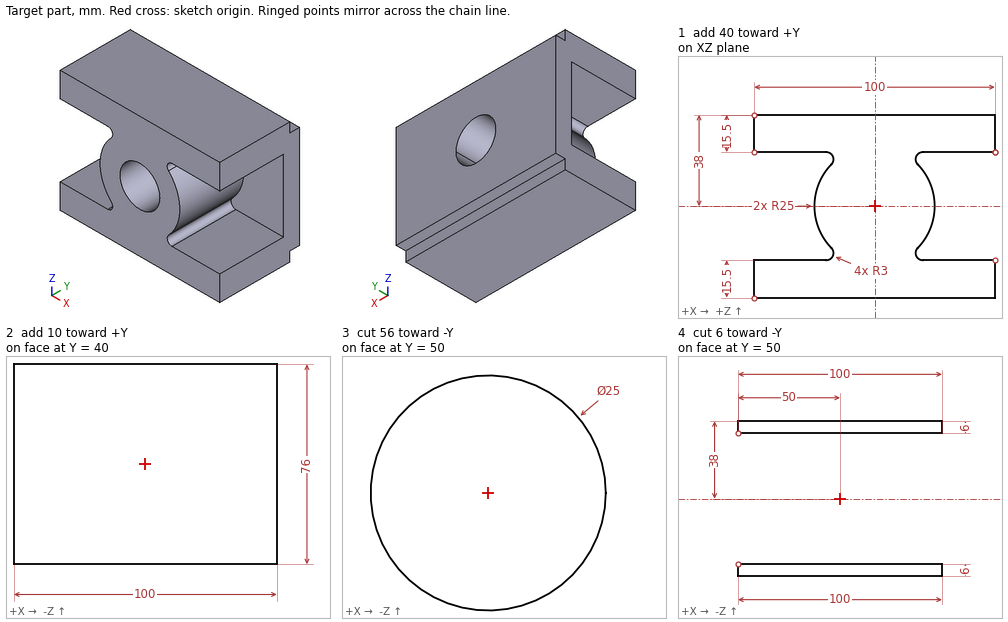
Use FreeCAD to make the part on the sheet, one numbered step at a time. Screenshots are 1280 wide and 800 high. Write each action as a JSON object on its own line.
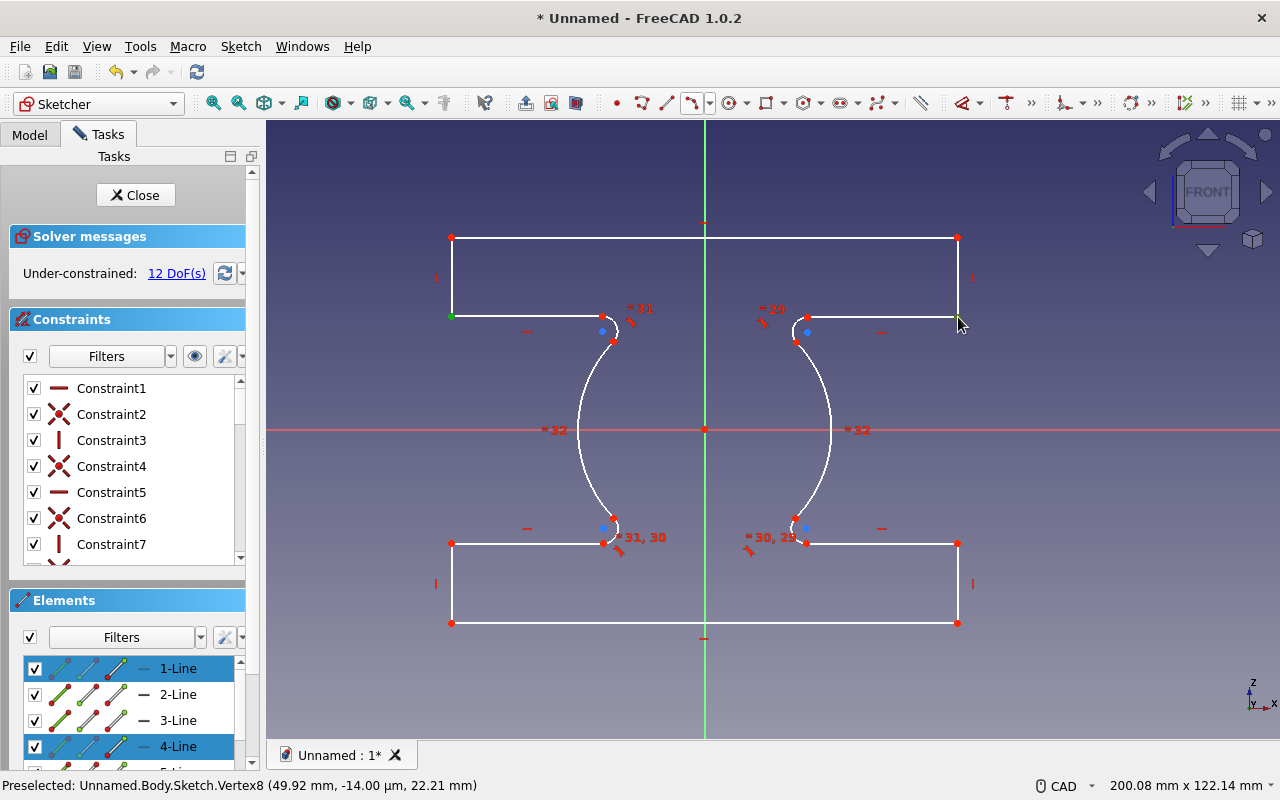
{"action": "left_click", "coordinate": [705, 671]}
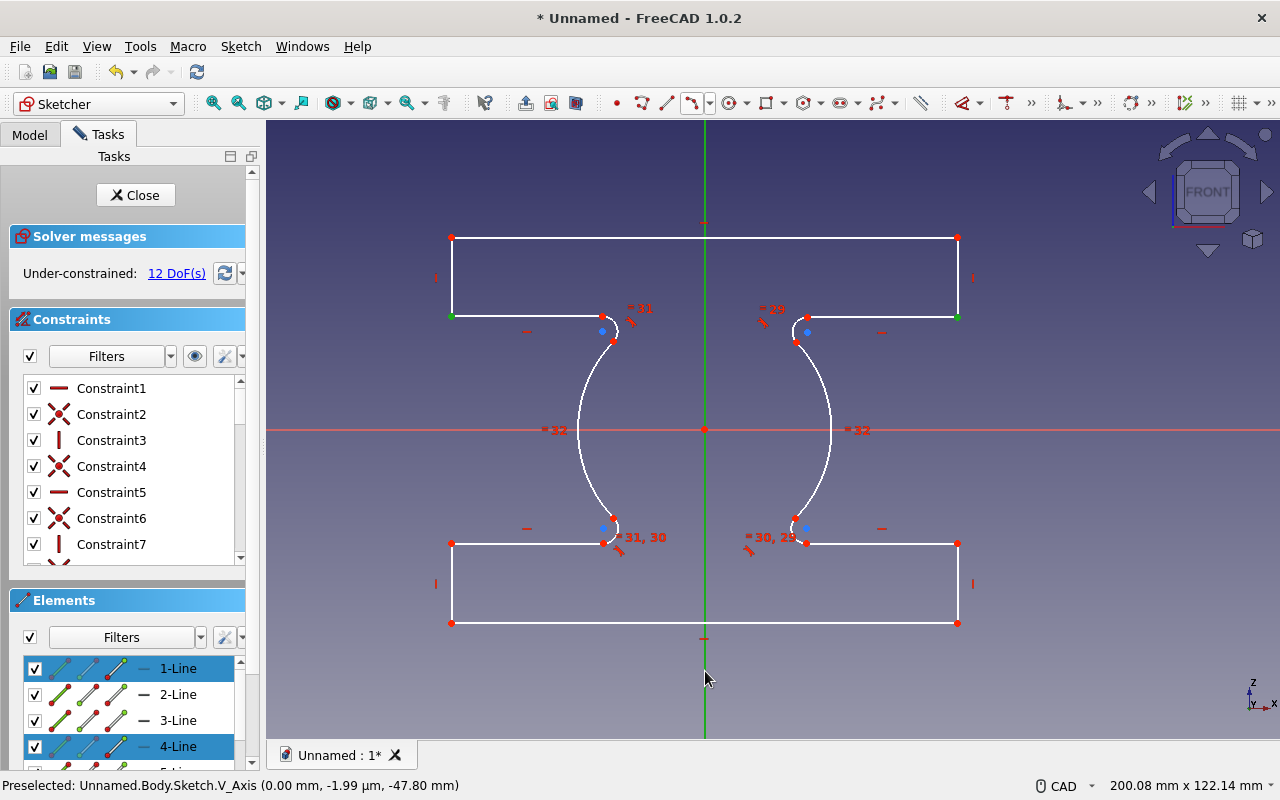
{"action": "key", "text": "s"}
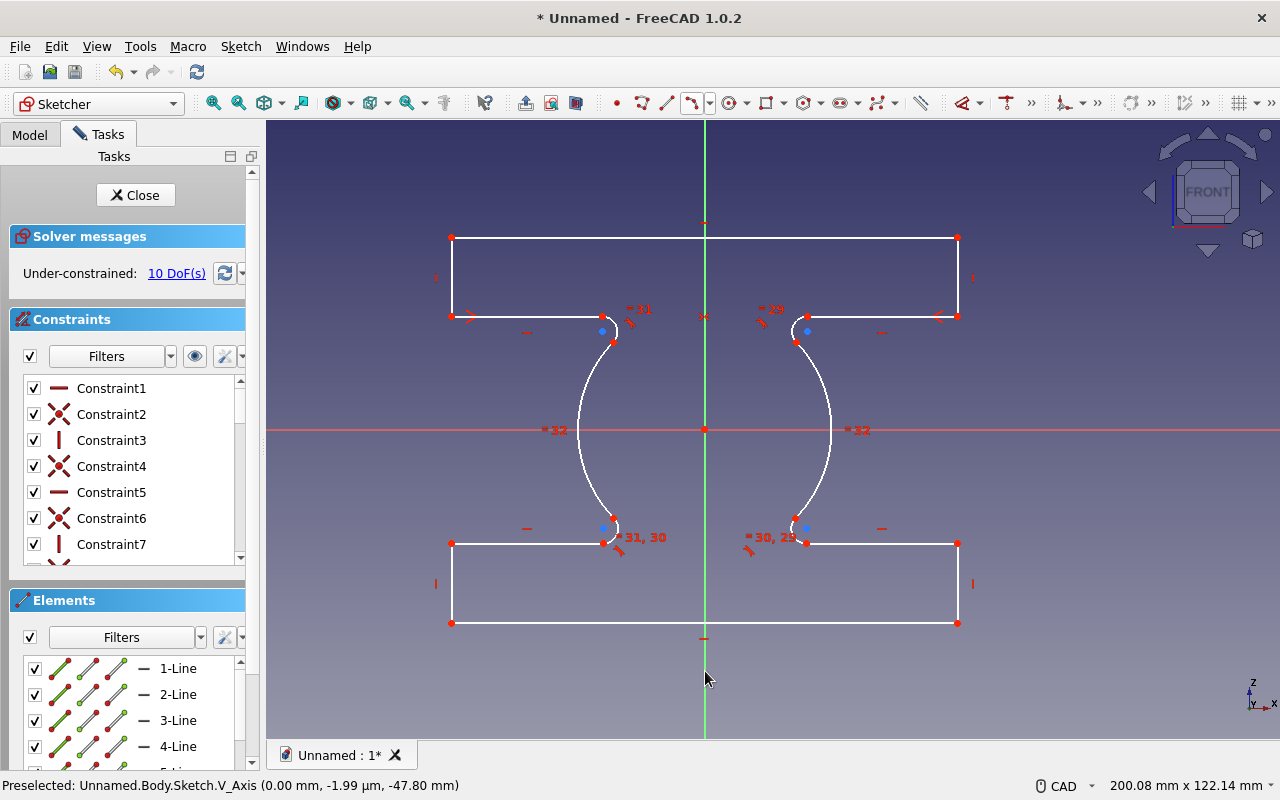
{"action": "left_click", "coordinate": [958, 317]}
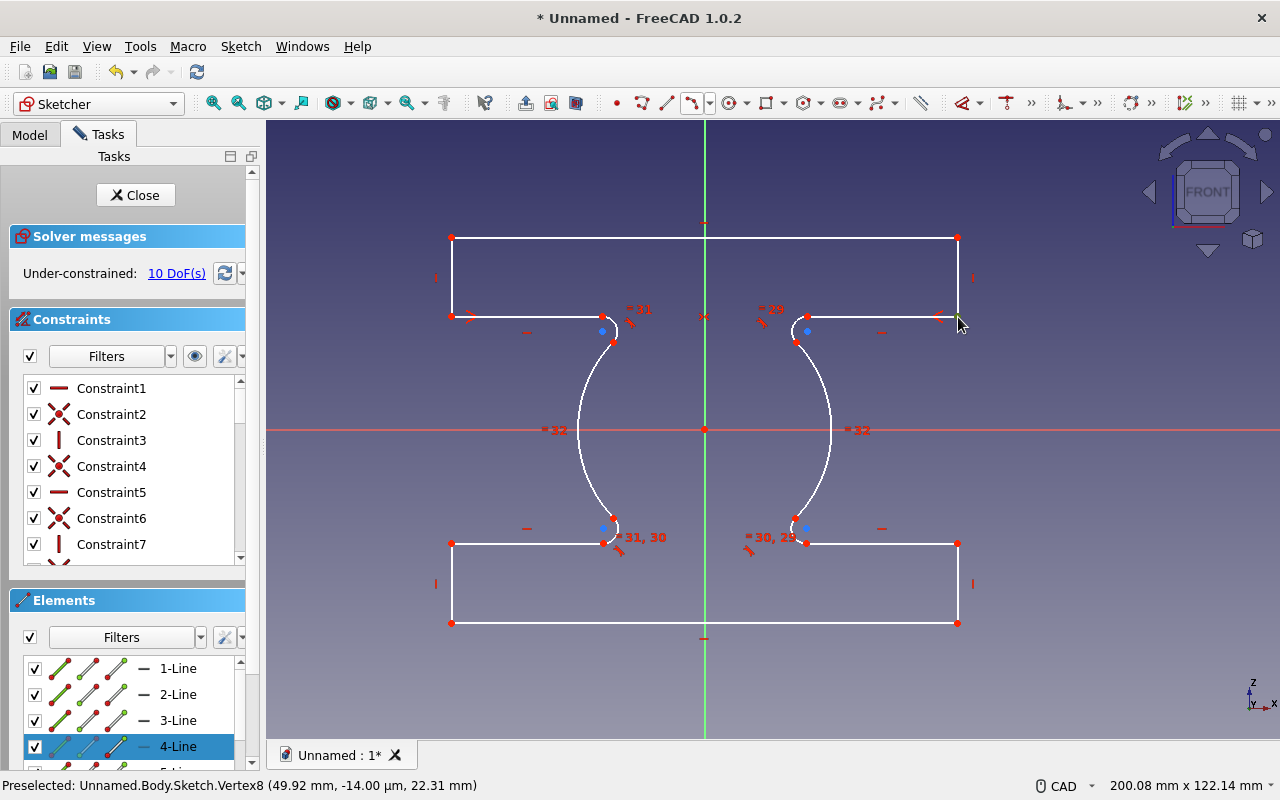
{"action": "left_click", "coordinate": [958, 544]}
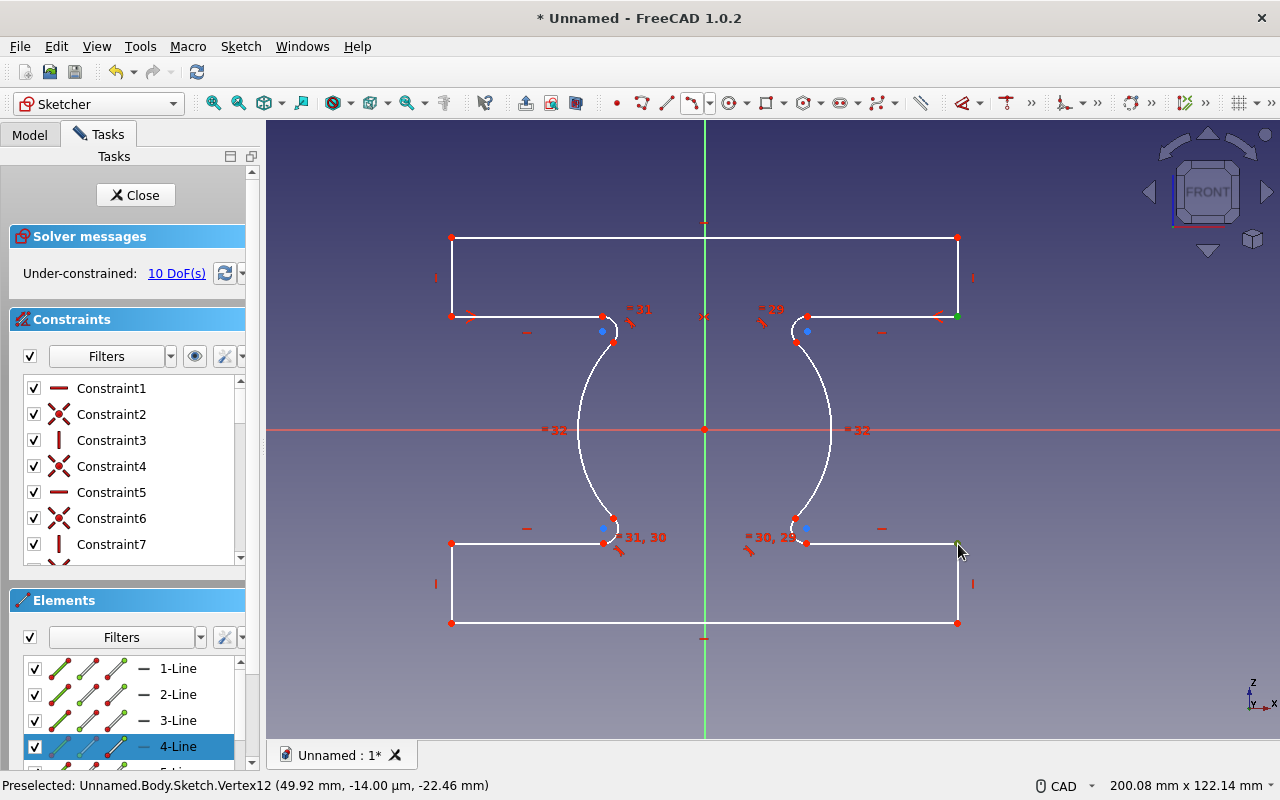
{"action": "left_click", "coordinate": [353, 430]}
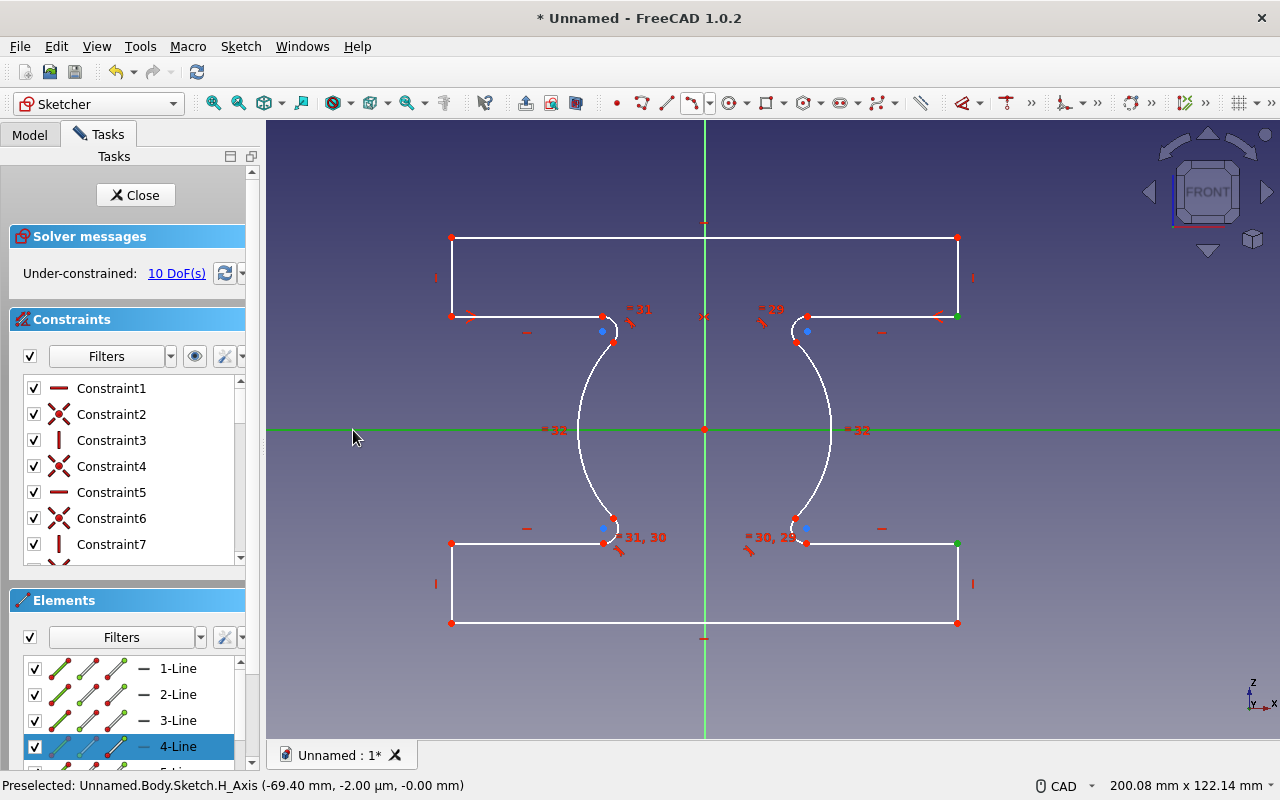
{"action": "key", "text": "s"}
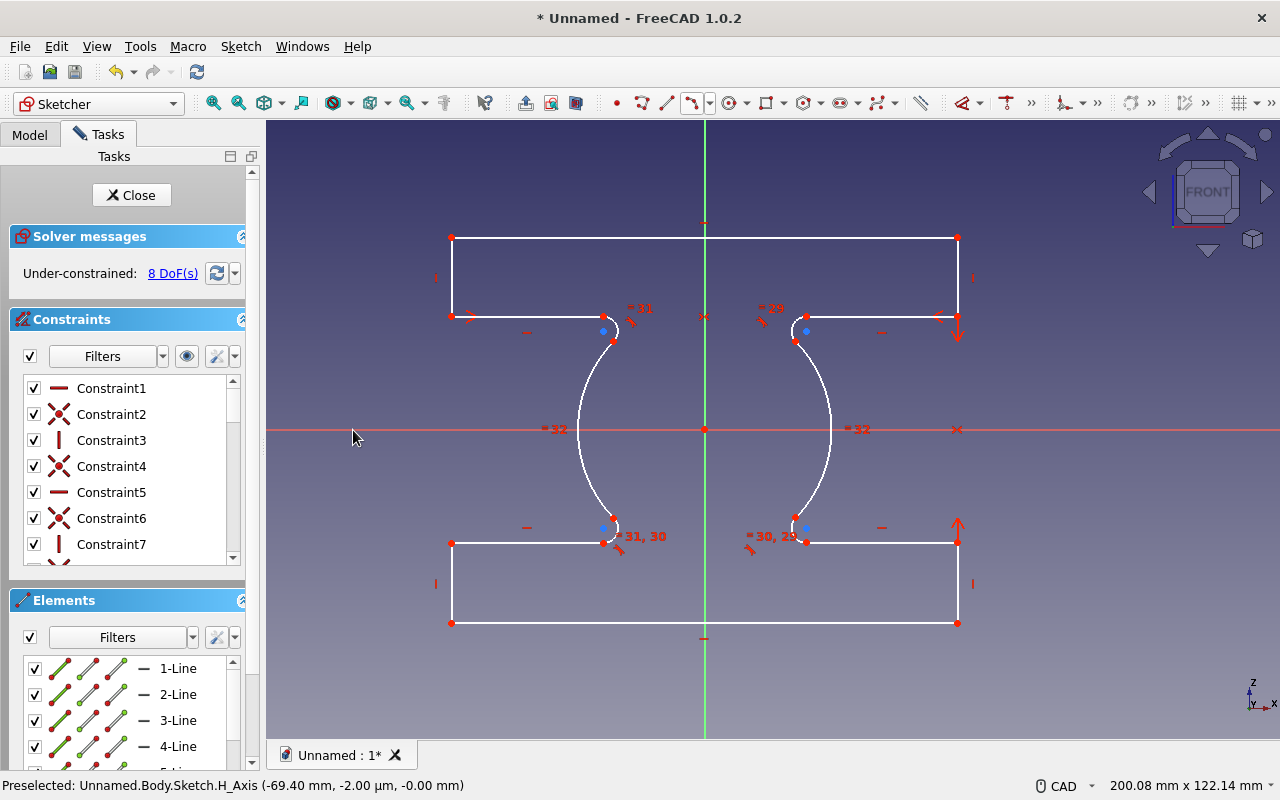
{"action": "left_click", "coordinate": [452, 238]}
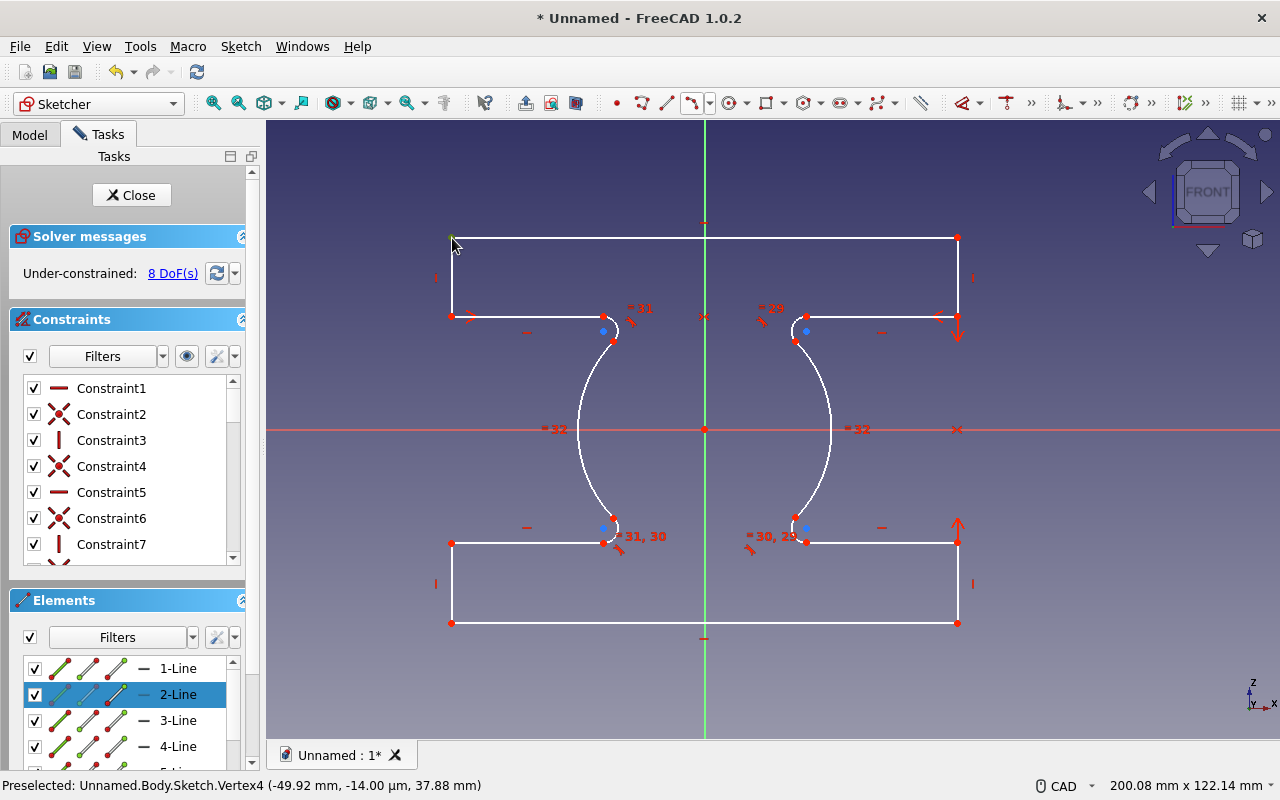
{"action": "left_click", "coordinate": [452, 623]}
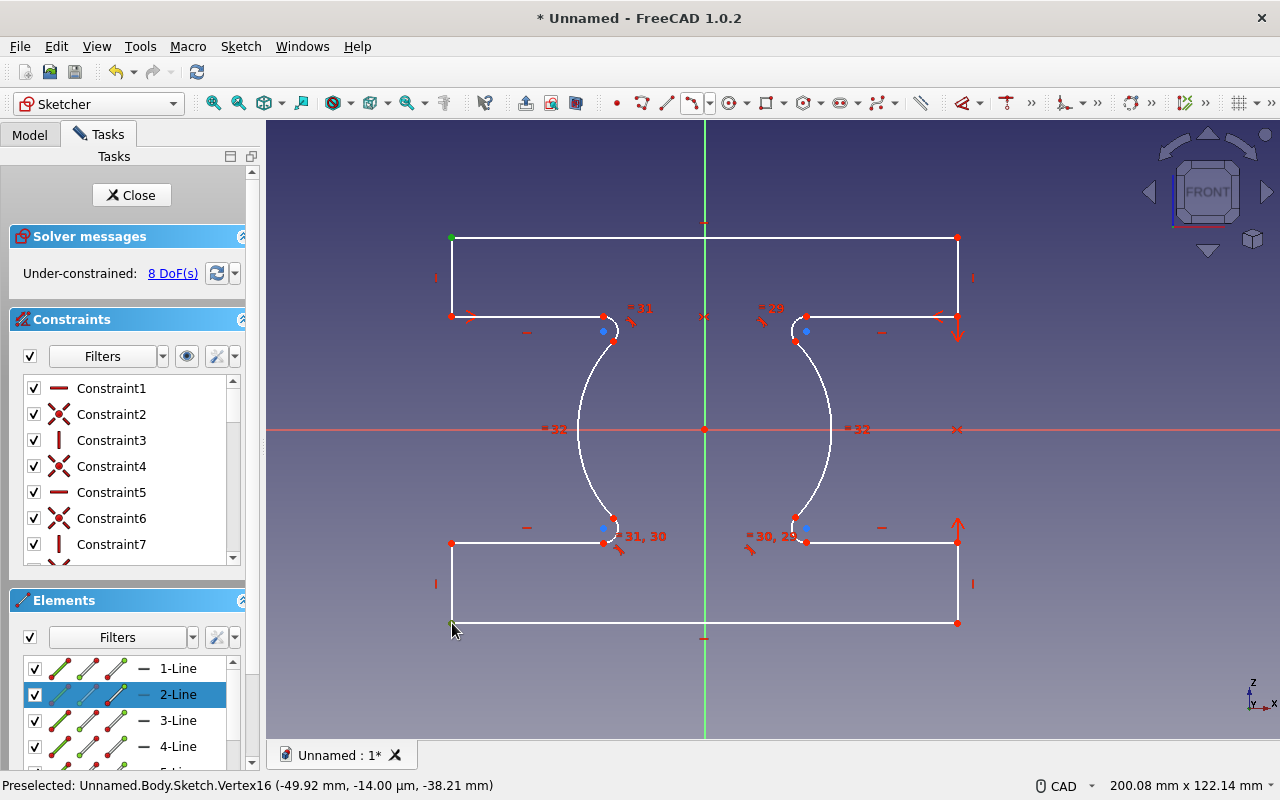
{"action": "left_click", "coordinate": [353, 430]}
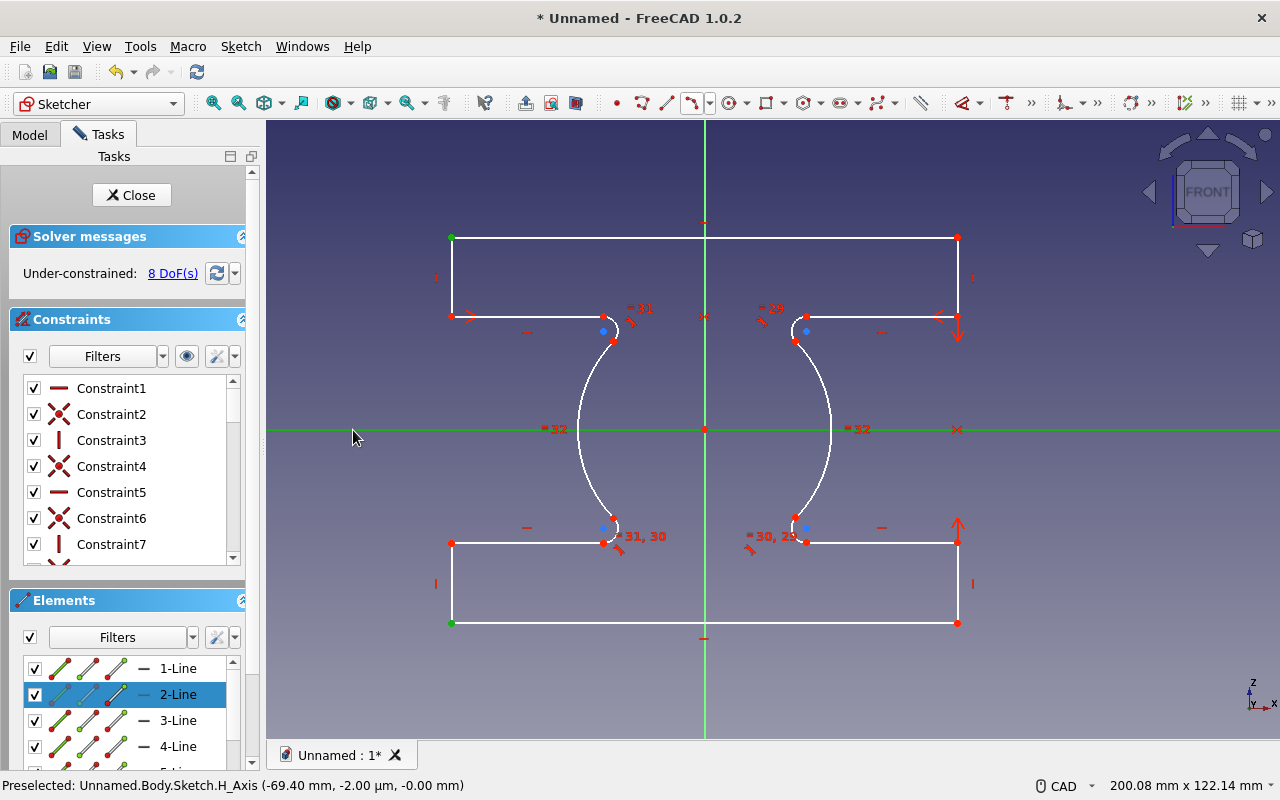
{"action": "key", "text": "s"}